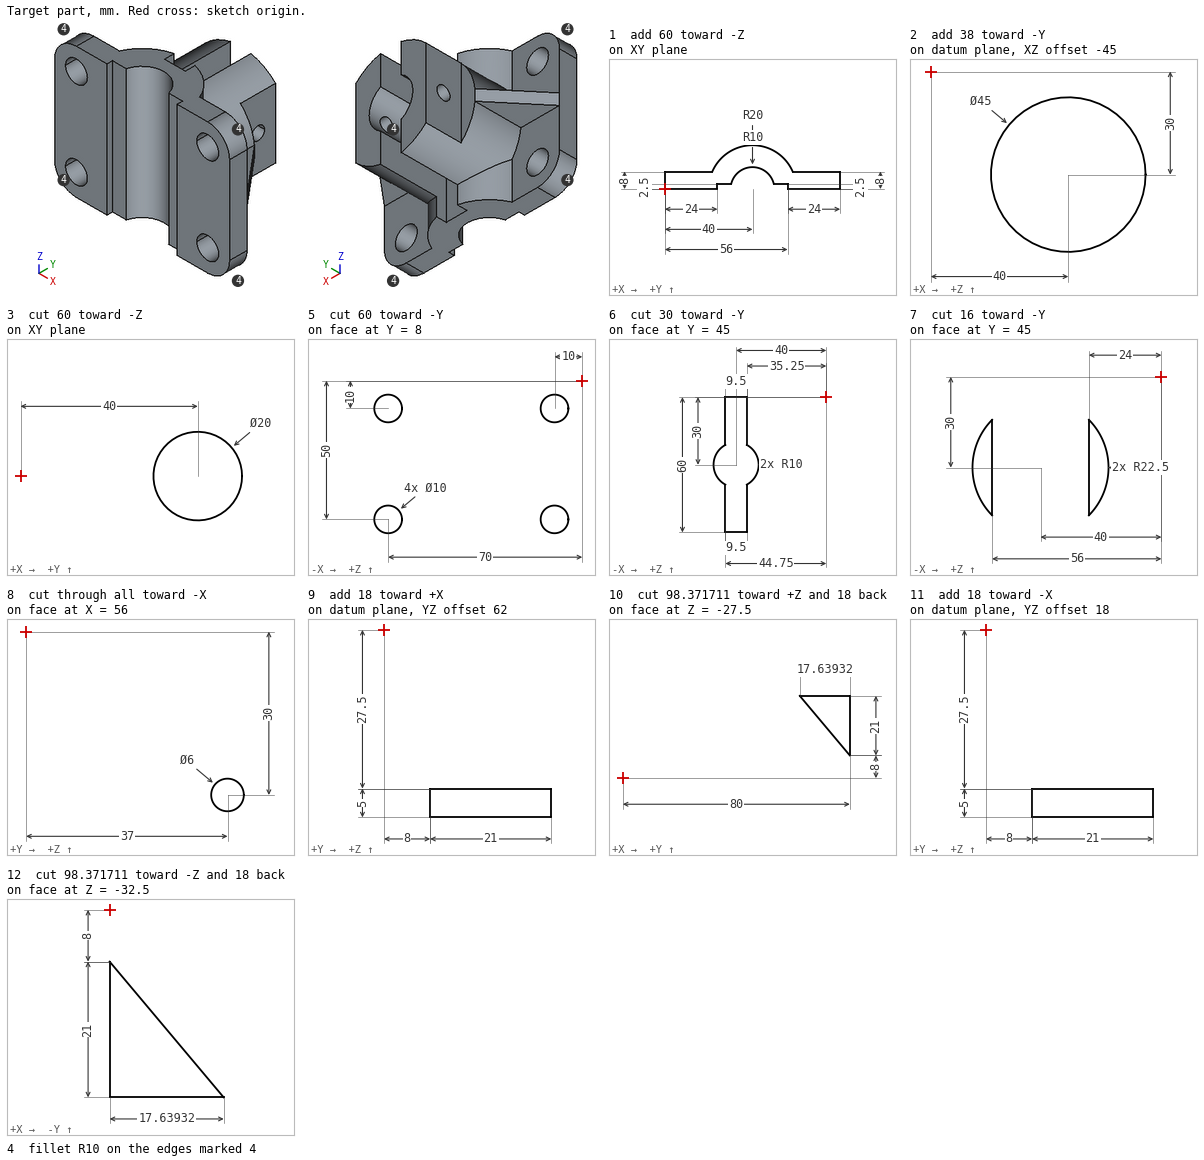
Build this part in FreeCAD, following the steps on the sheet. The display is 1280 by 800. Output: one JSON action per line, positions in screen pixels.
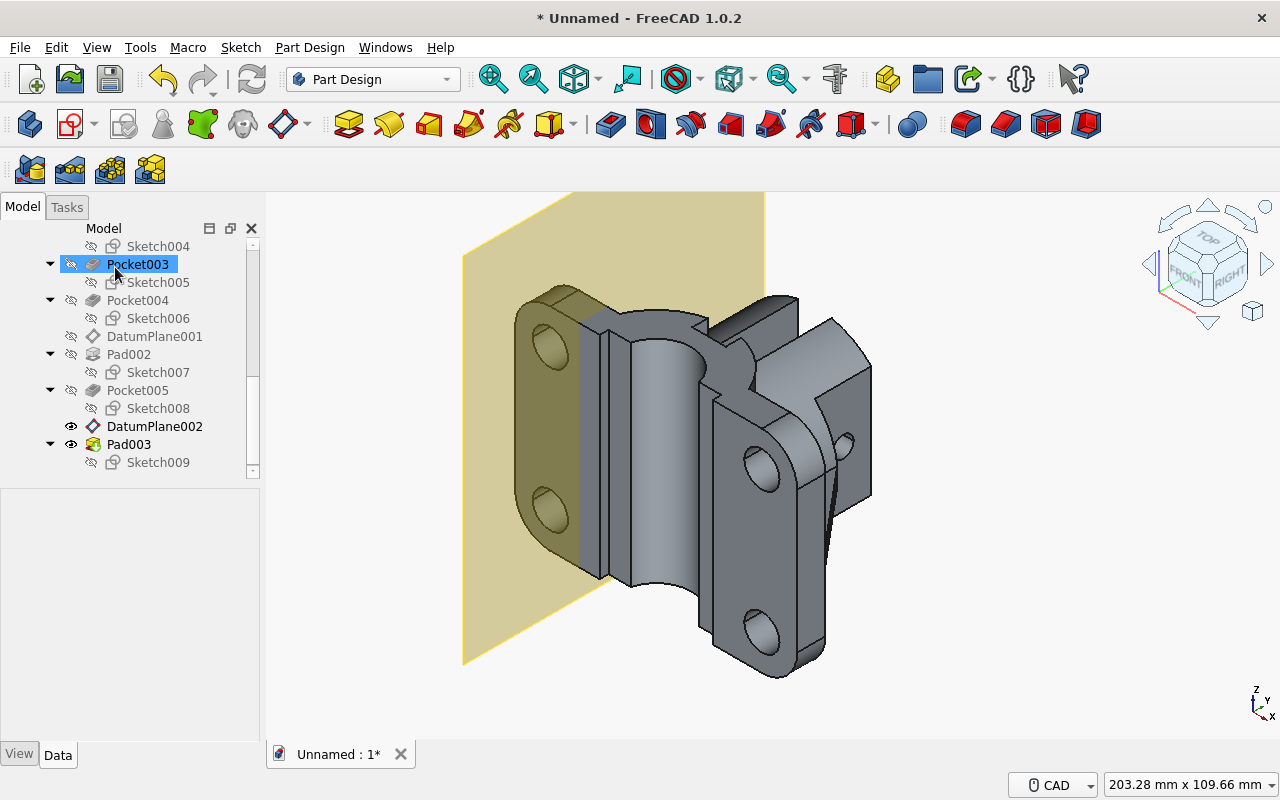
{"action": "left_click", "coordinate": [116, 426]}
{"action": "key", "text": "space"}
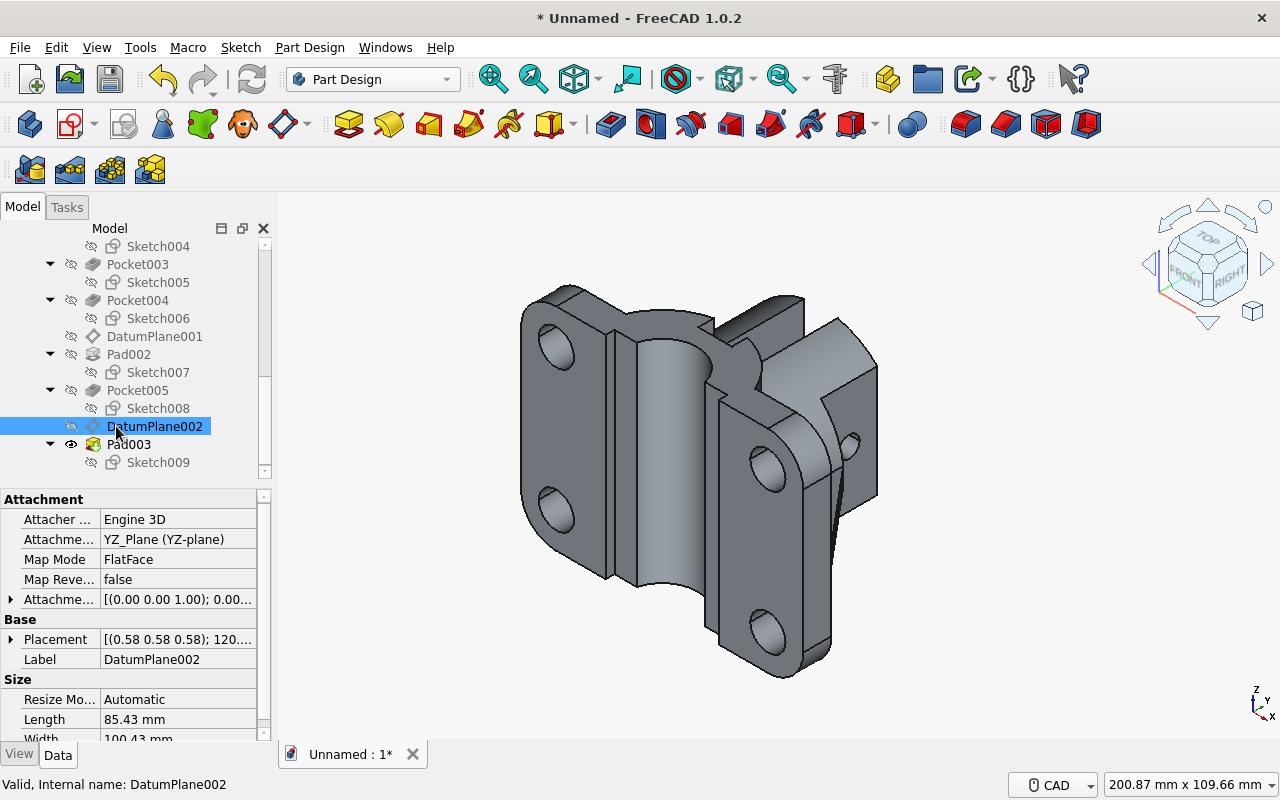
{"action": "key", "text": "5"}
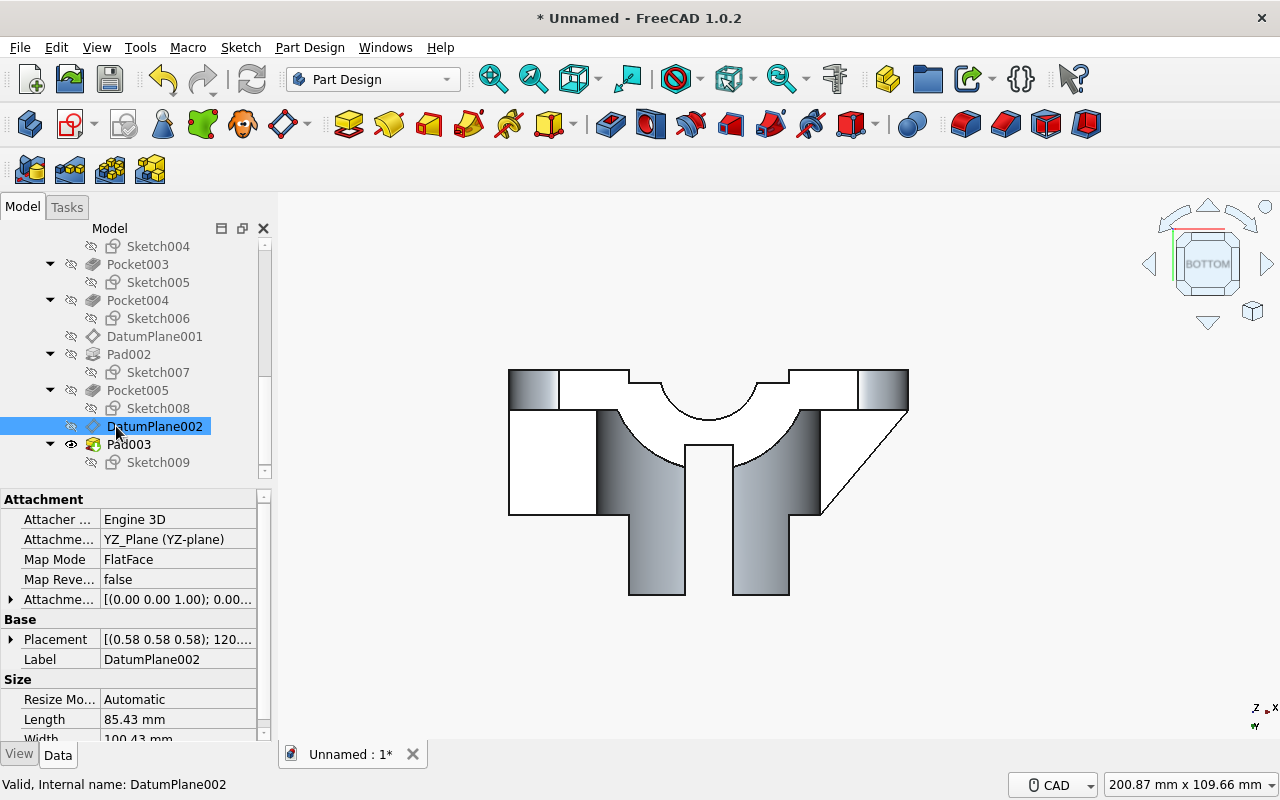
{"action": "left_click", "coordinate": [494, 80]}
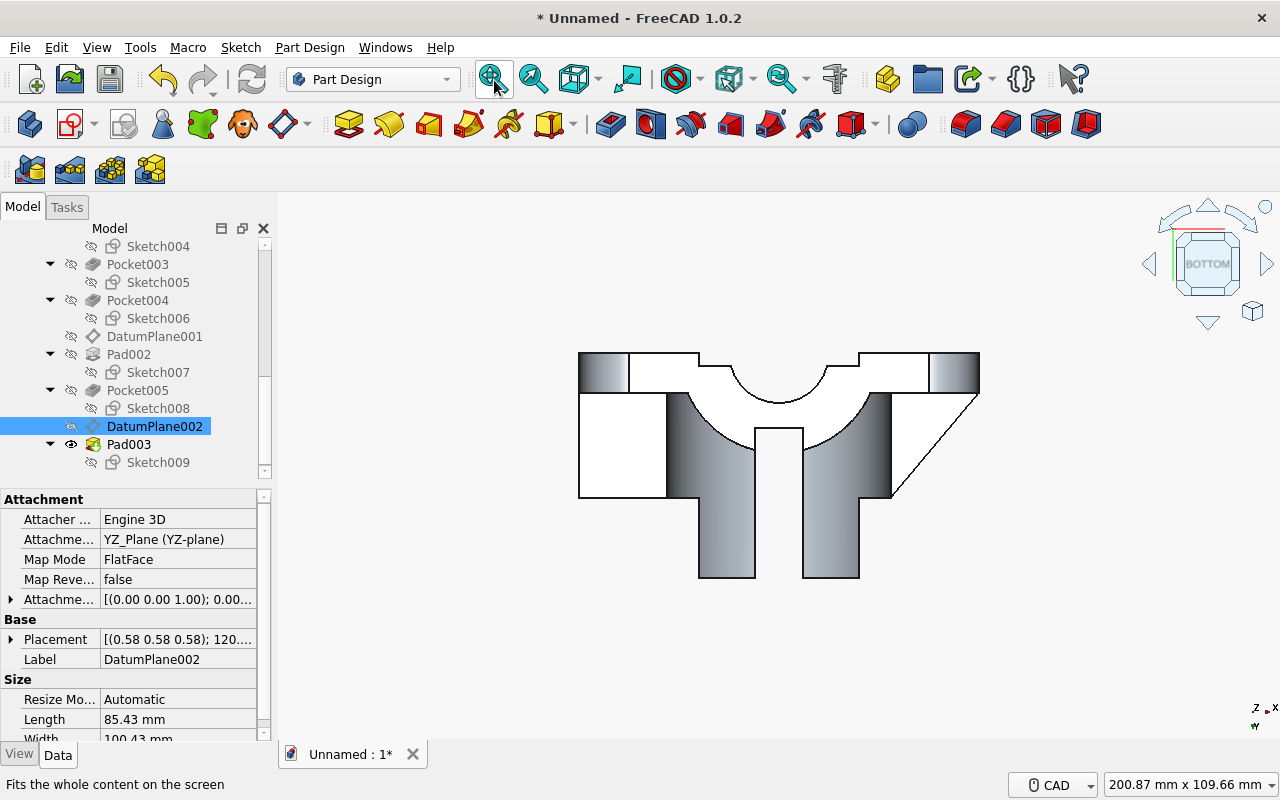
{"action": "left_click", "coordinate": [623, 445]}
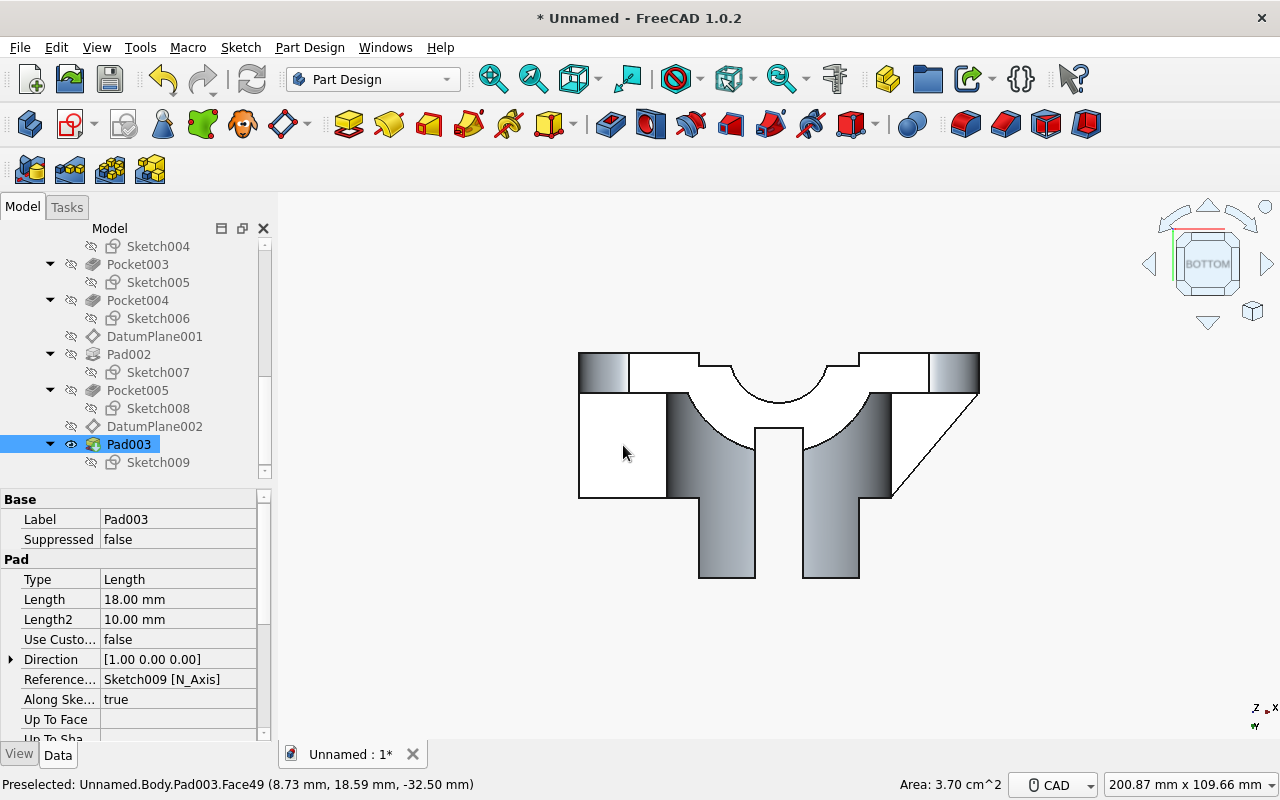
{"action": "left_click", "coordinate": [70, 124]}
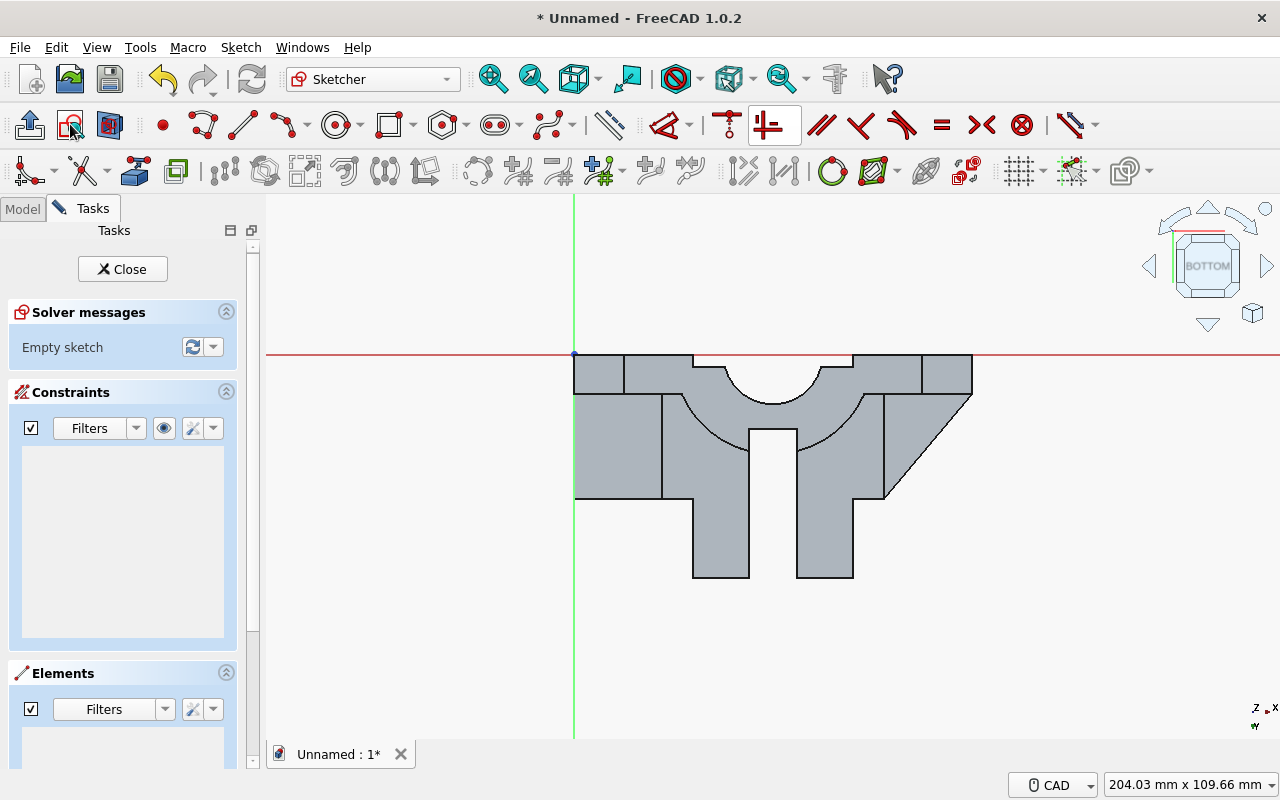
{"action": "scroll", "coordinate": [547, 394], "scroll_direction": "up", "scroll_amount": 4}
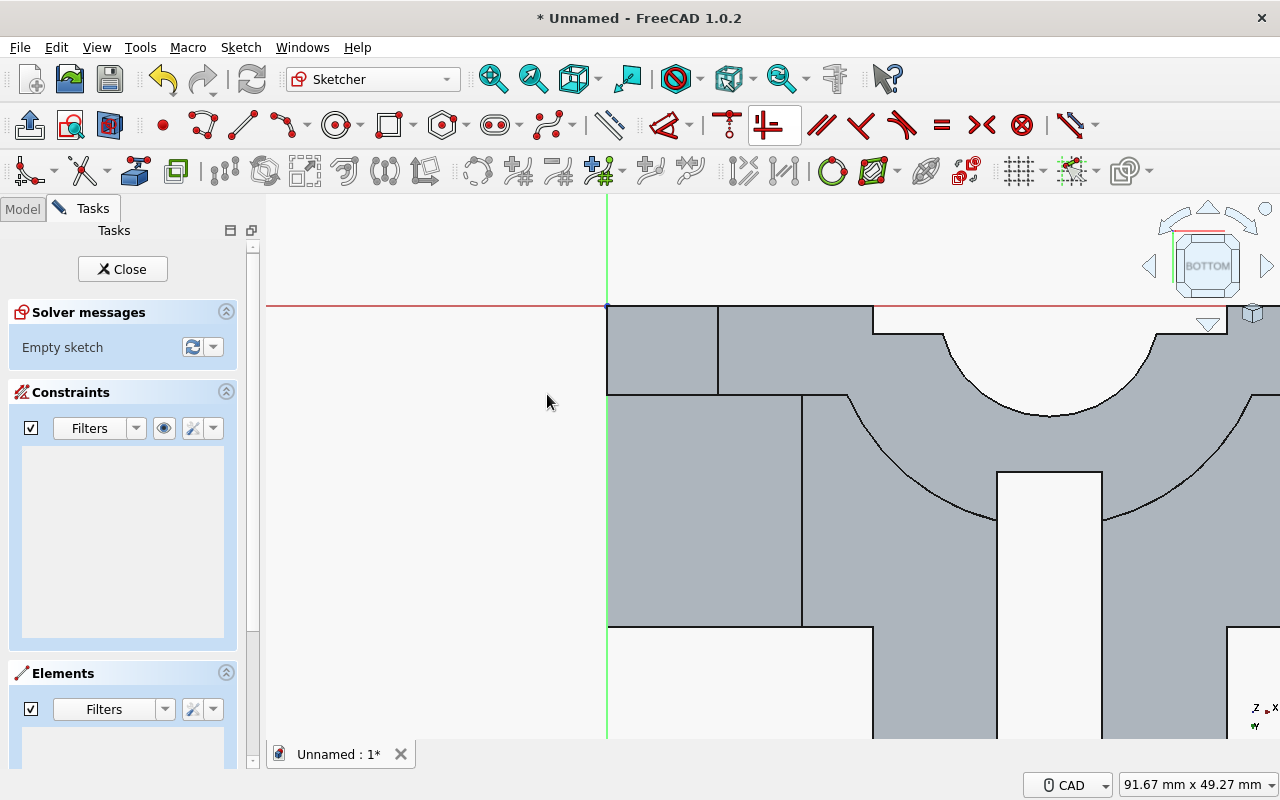
{"action": "left_click", "coordinate": [204, 126]}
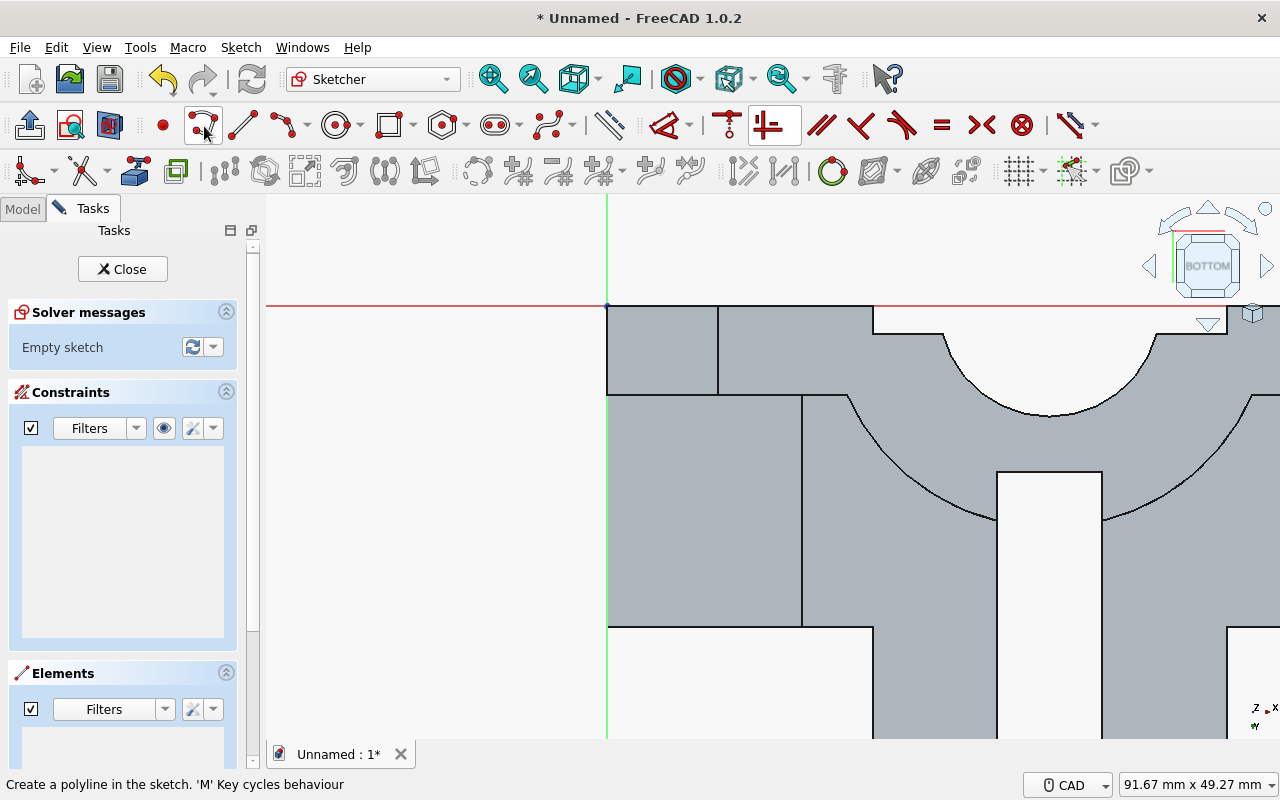
{"action": "left_click", "coordinate": [607, 395]}
{"action": "left_click", "coordinate": [616, 627]}
{"action": "left_click", "coordinate": [802, 627]}
{"action": "left_click", "coordinate": [607, 396]}
{"action": "key", "text": "Escape"}
{"action": "key", "text": "Escape"}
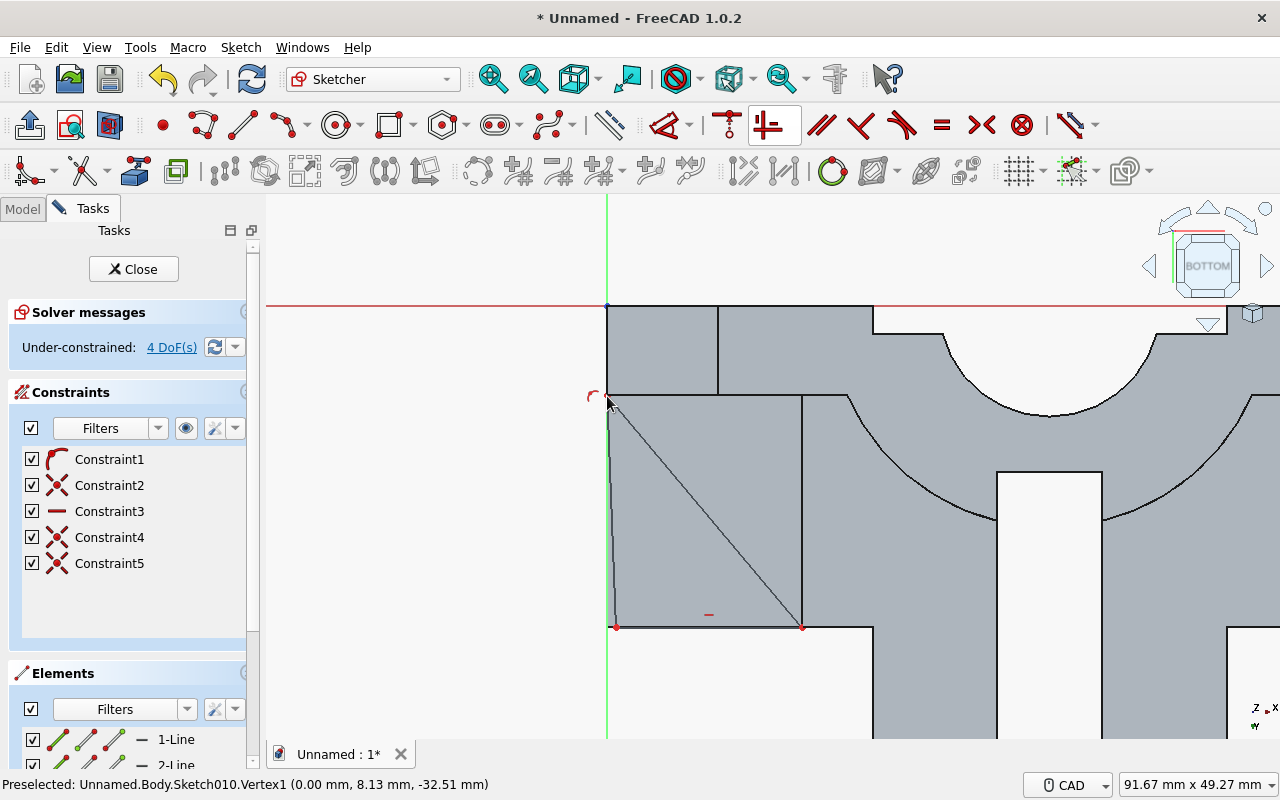
{"action": "left_click", "coordinate": [610, 466]}